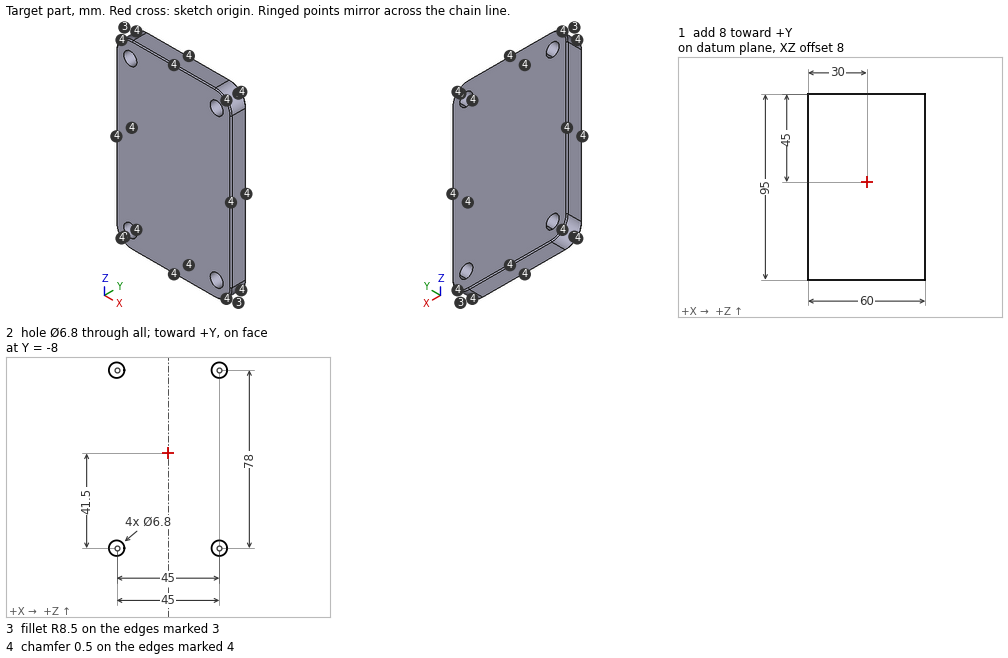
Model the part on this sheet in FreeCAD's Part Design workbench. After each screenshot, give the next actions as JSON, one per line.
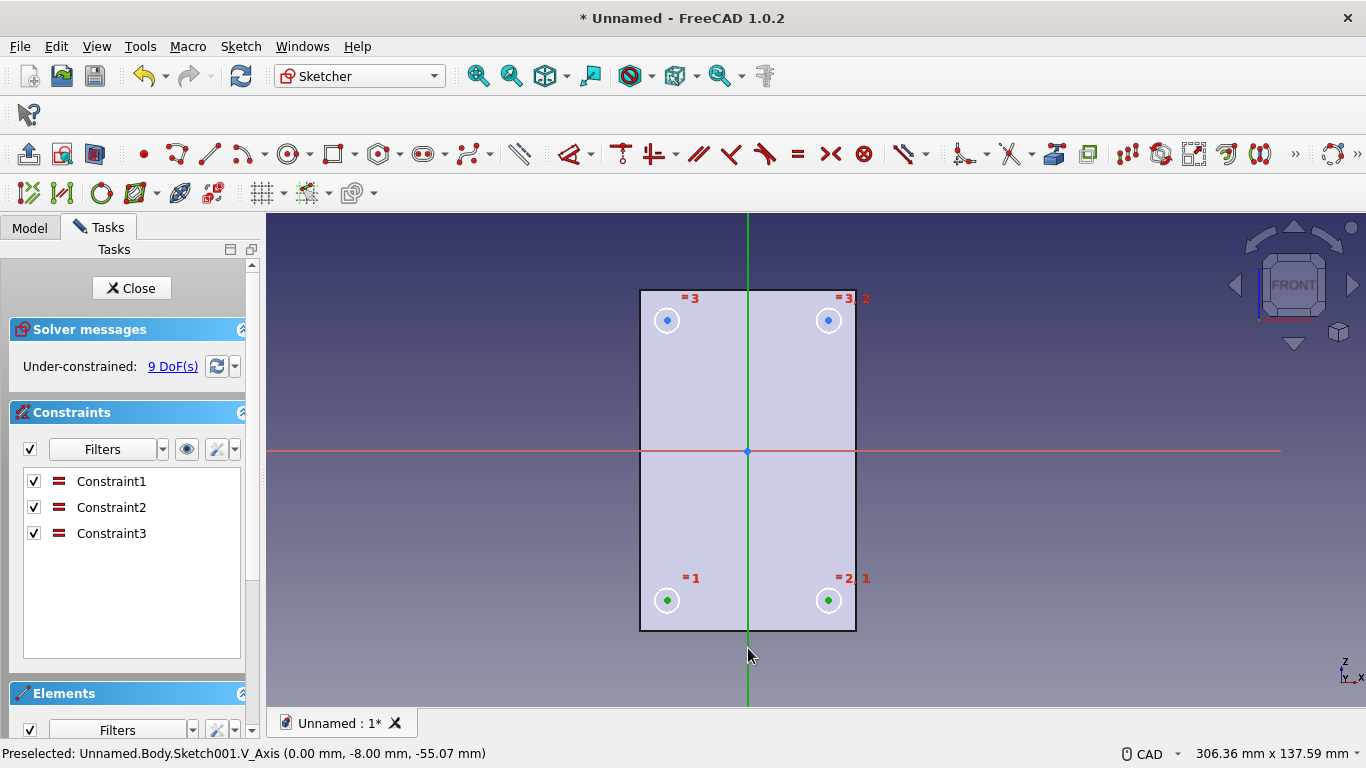
{"action": "key", "text": "s"}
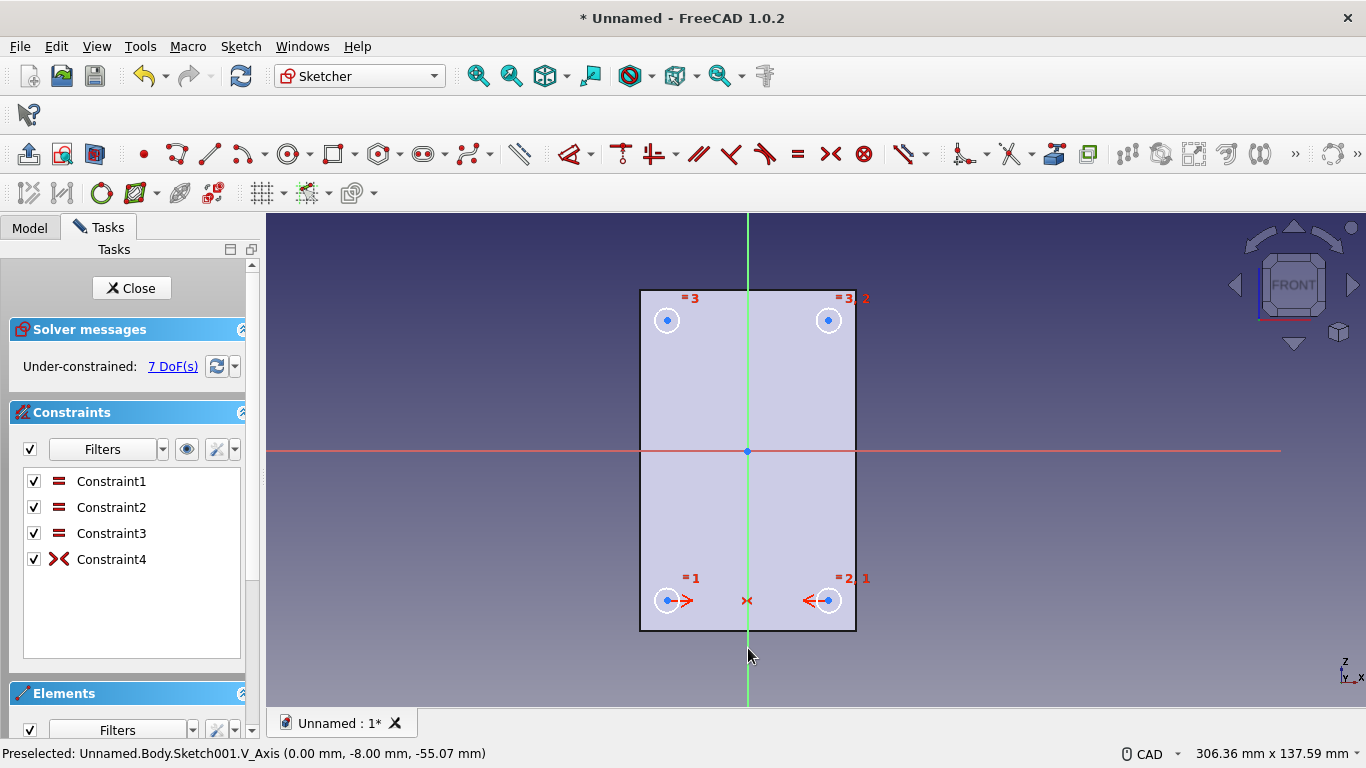
{"action": "left_click", "coordinate": [829, 321]}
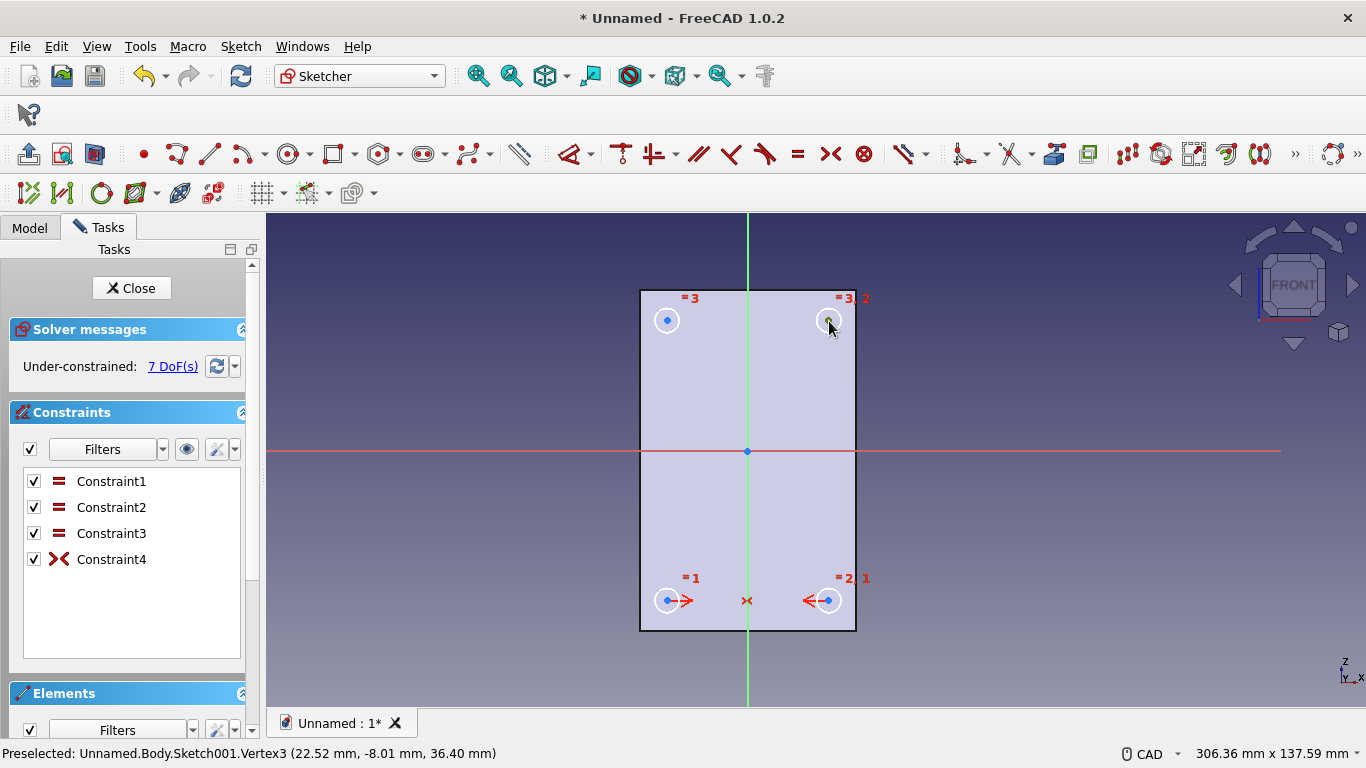
{"action": "left_click", "coordinate": [667, 321]}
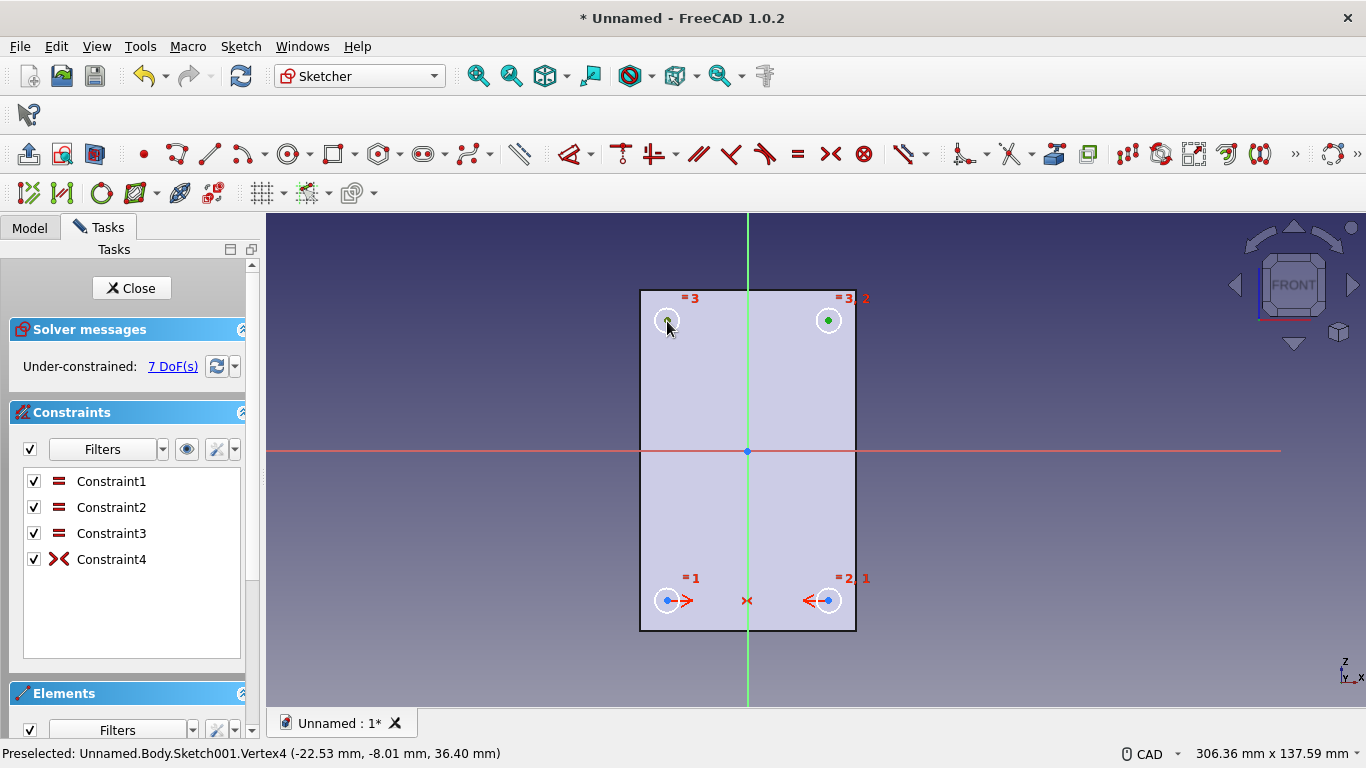
{"action": "left_click", "coordinate": [748, 648]}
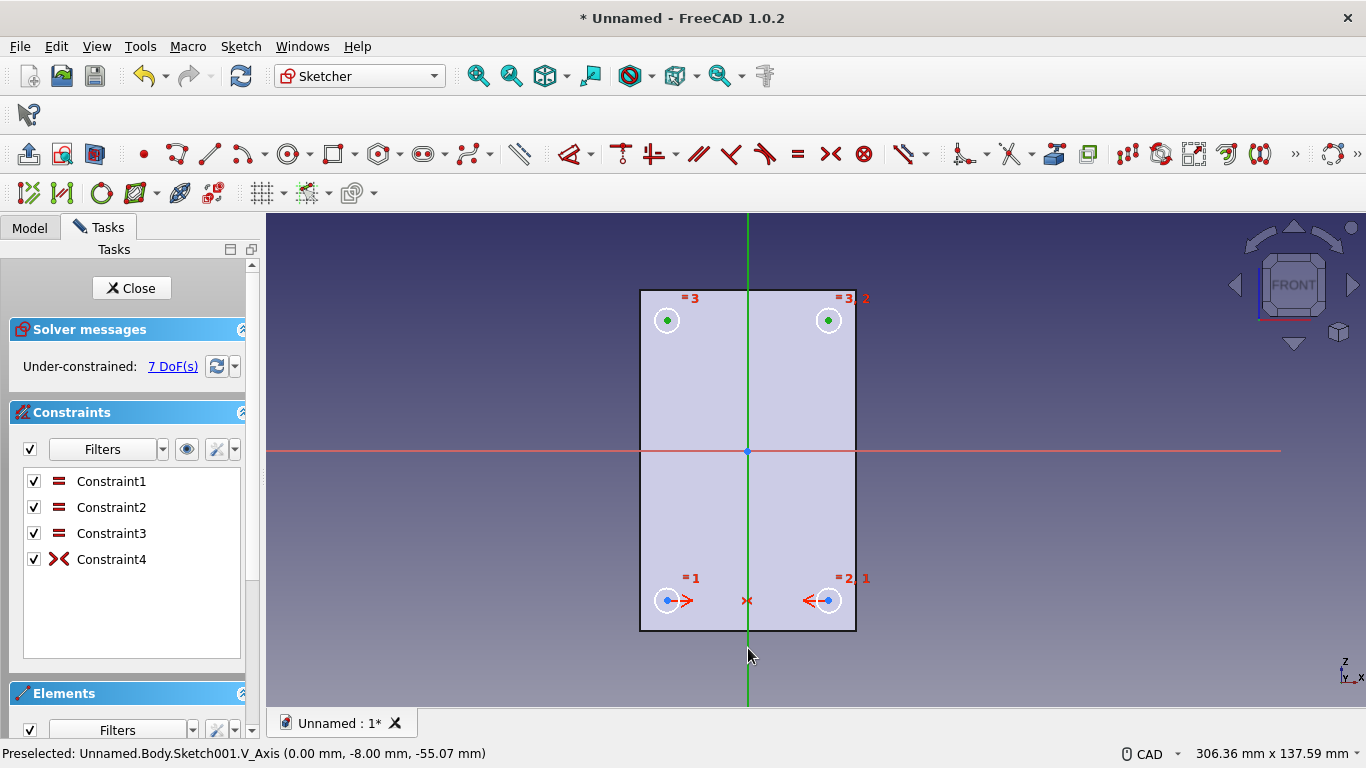
{"action": "left_click", "coordinate": [831, 154]}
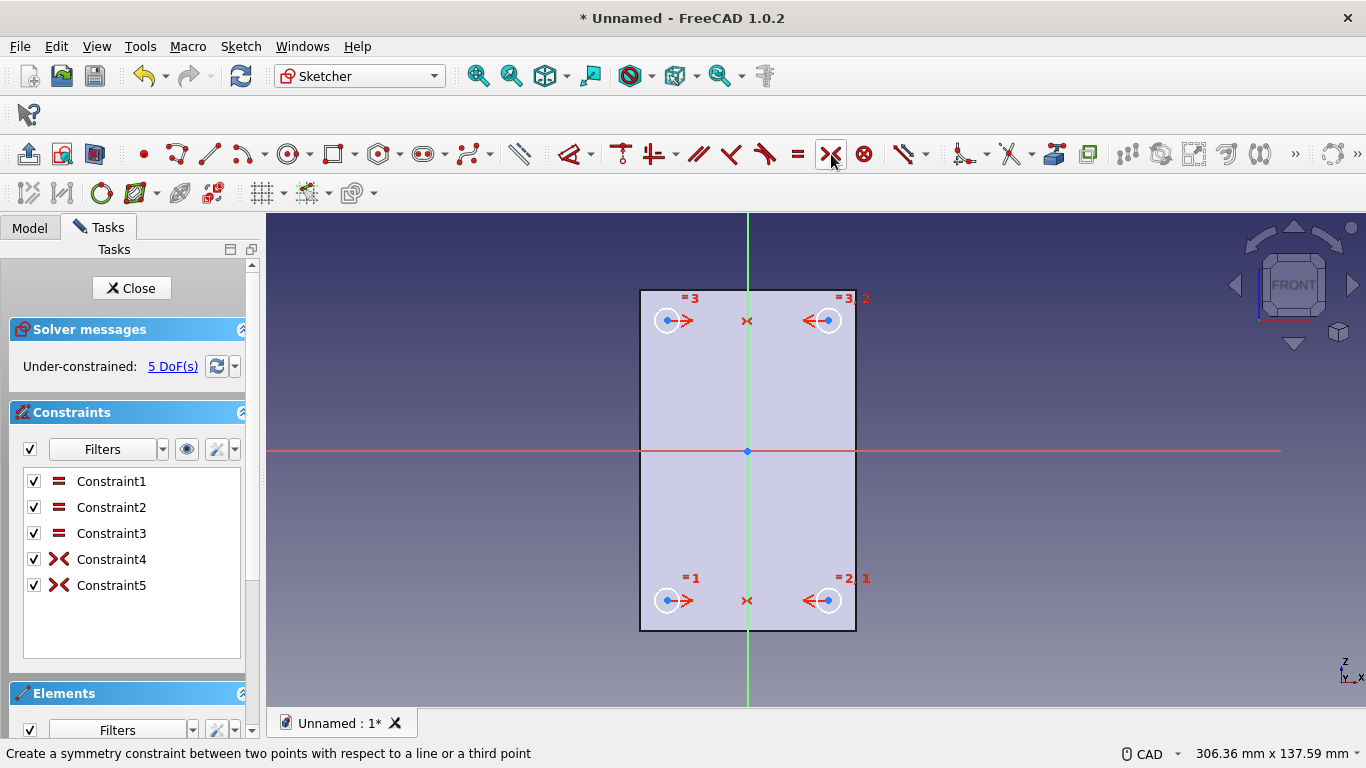
{"action": "left_click", "coordinate": [568, 154]}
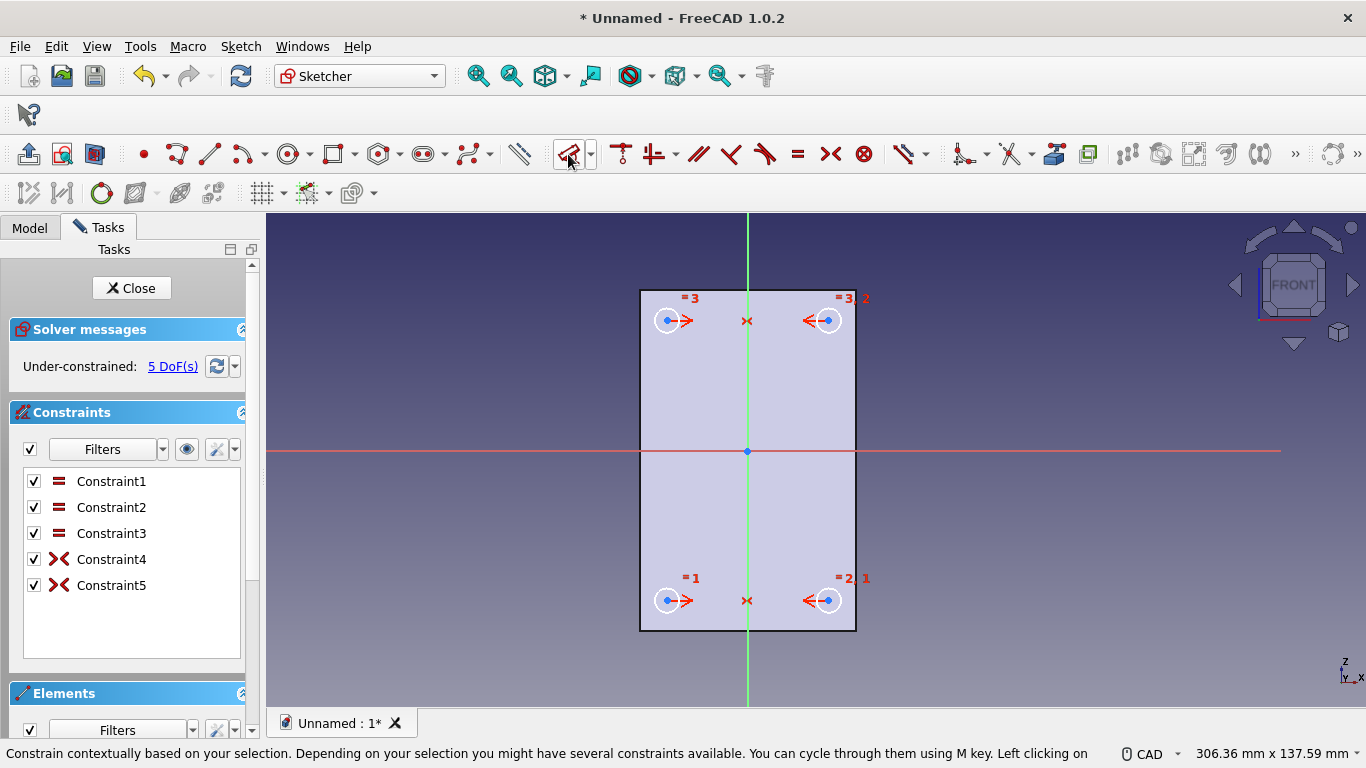
{"action": "scroll", "coordinate": [676, 592], "scroll_direction": "up", "scroll_amount": 3}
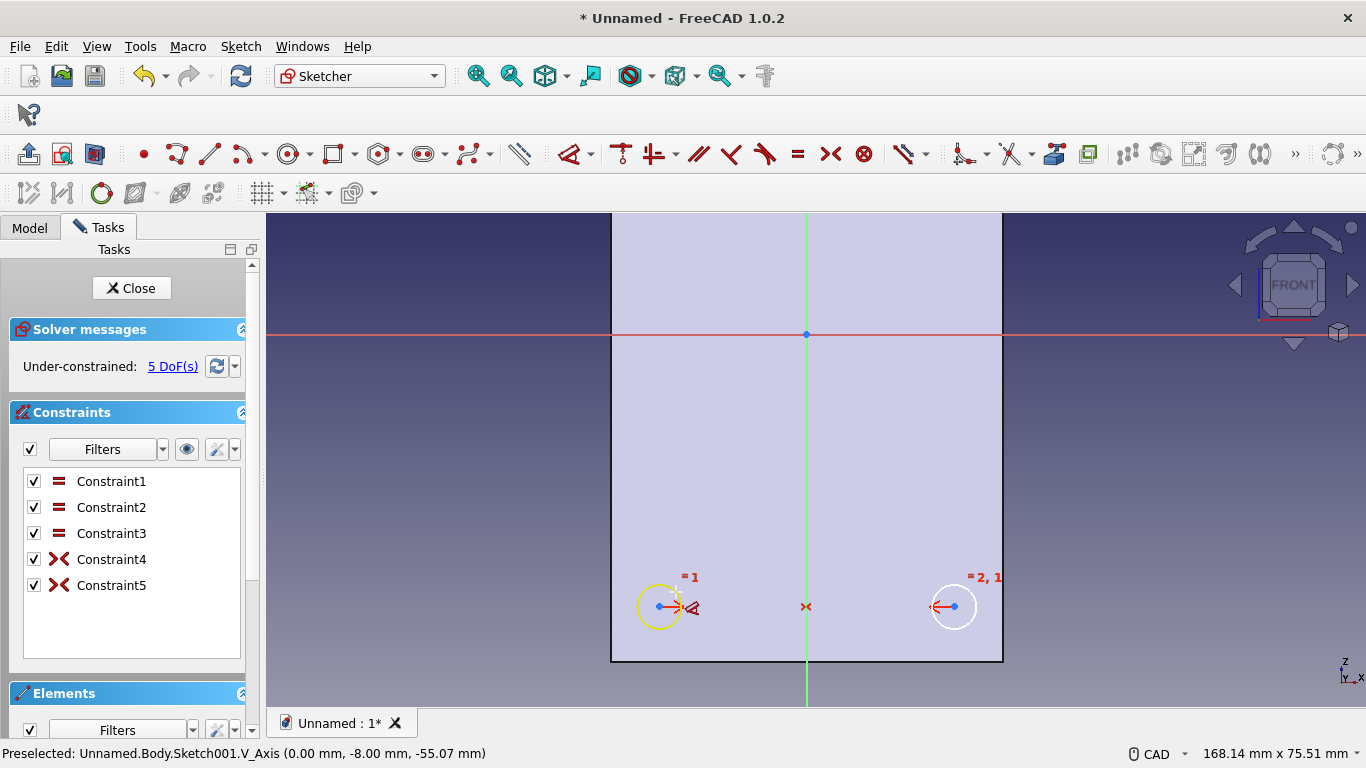
{"action": "left_click", "coordinate": [675, 591]}
{"action": "left_click", "coordinate": [697, 568]}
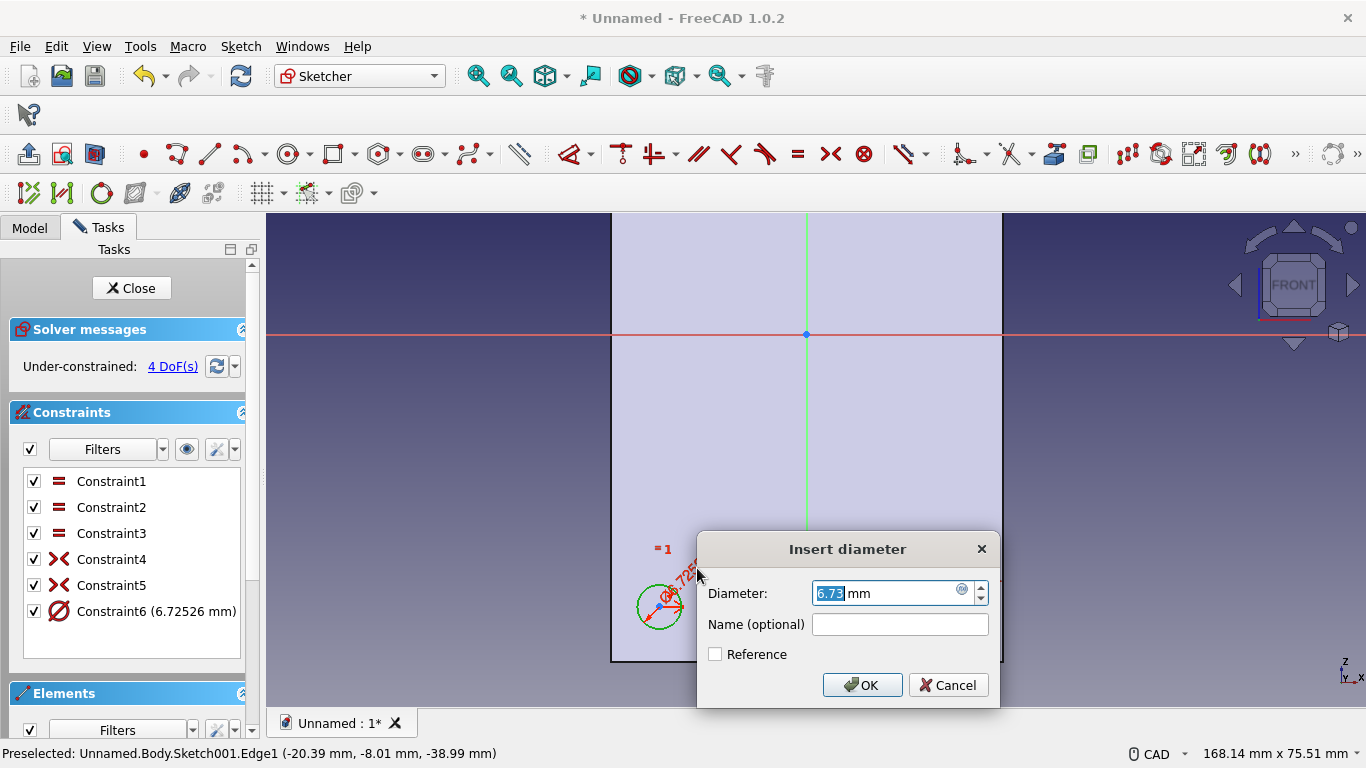
{"action": "type", "text": "6.8"}
{"action": "key", "text": "Return"}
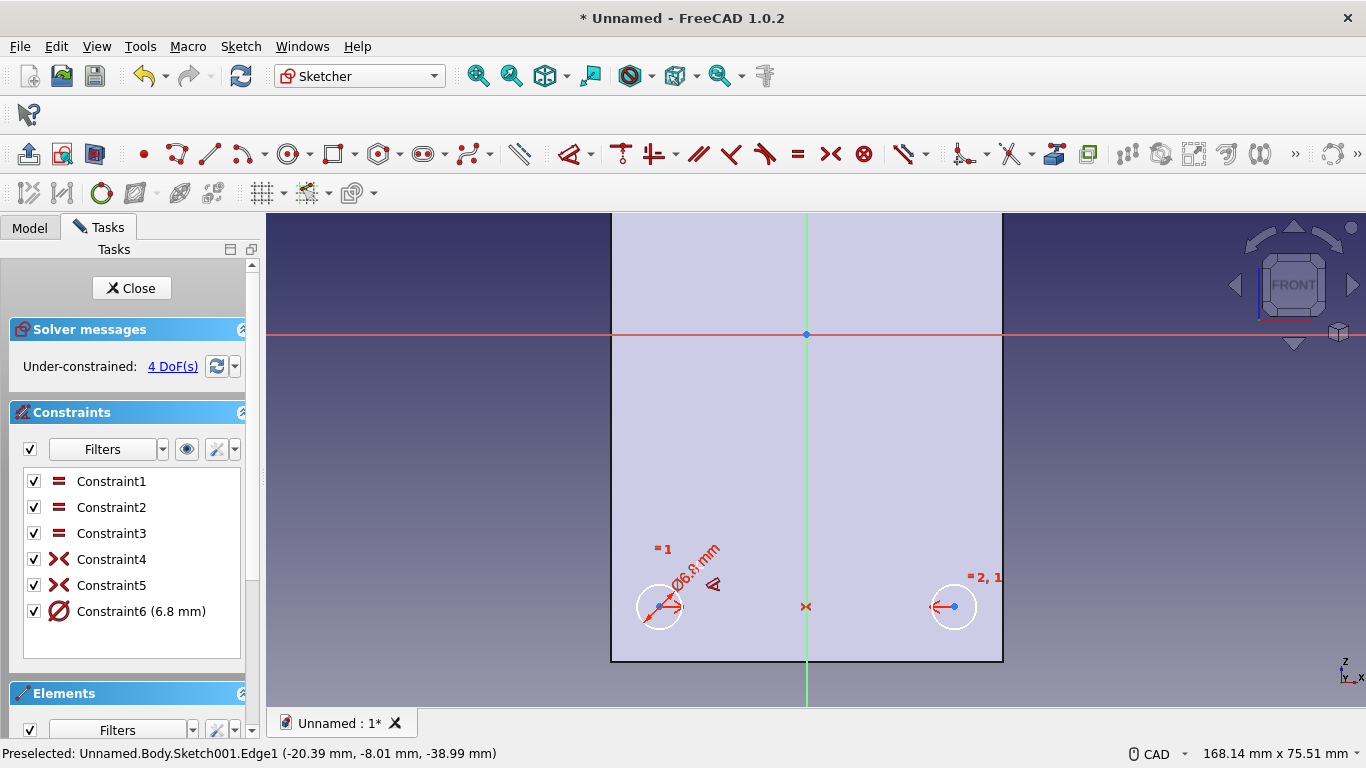
{"action": "left_click", "coordinate": [659, 607]}